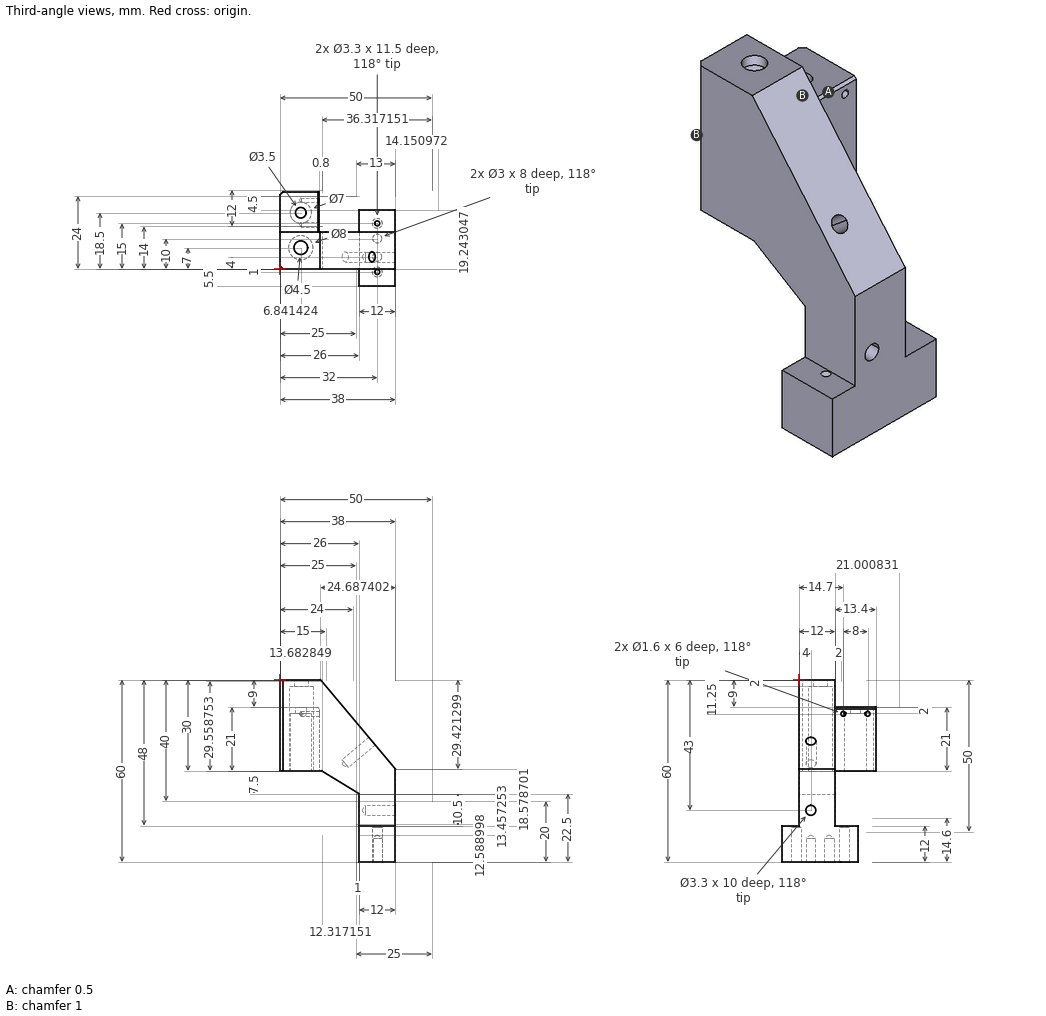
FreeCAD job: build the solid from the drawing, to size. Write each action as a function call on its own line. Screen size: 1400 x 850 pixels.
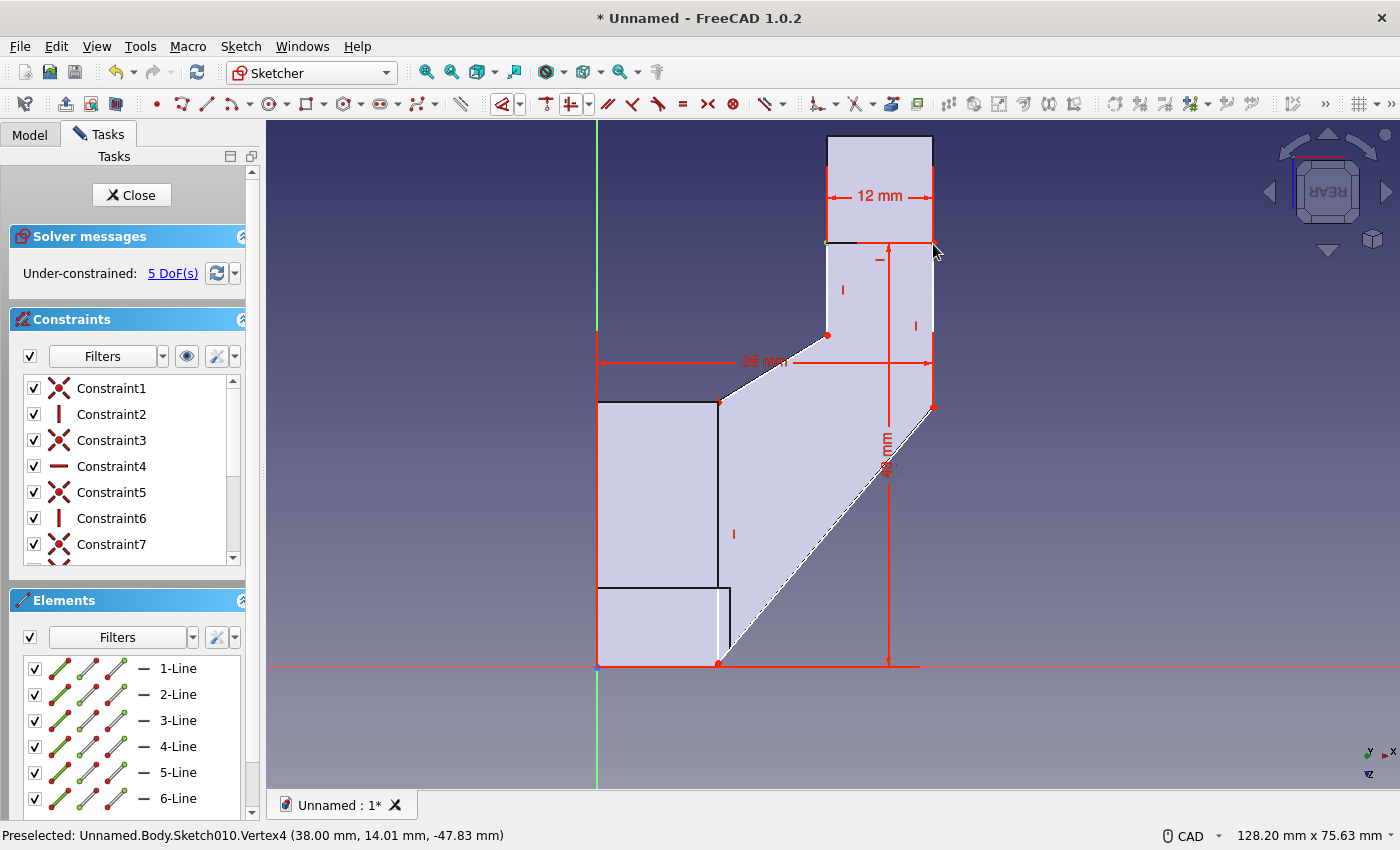
click(718, 403)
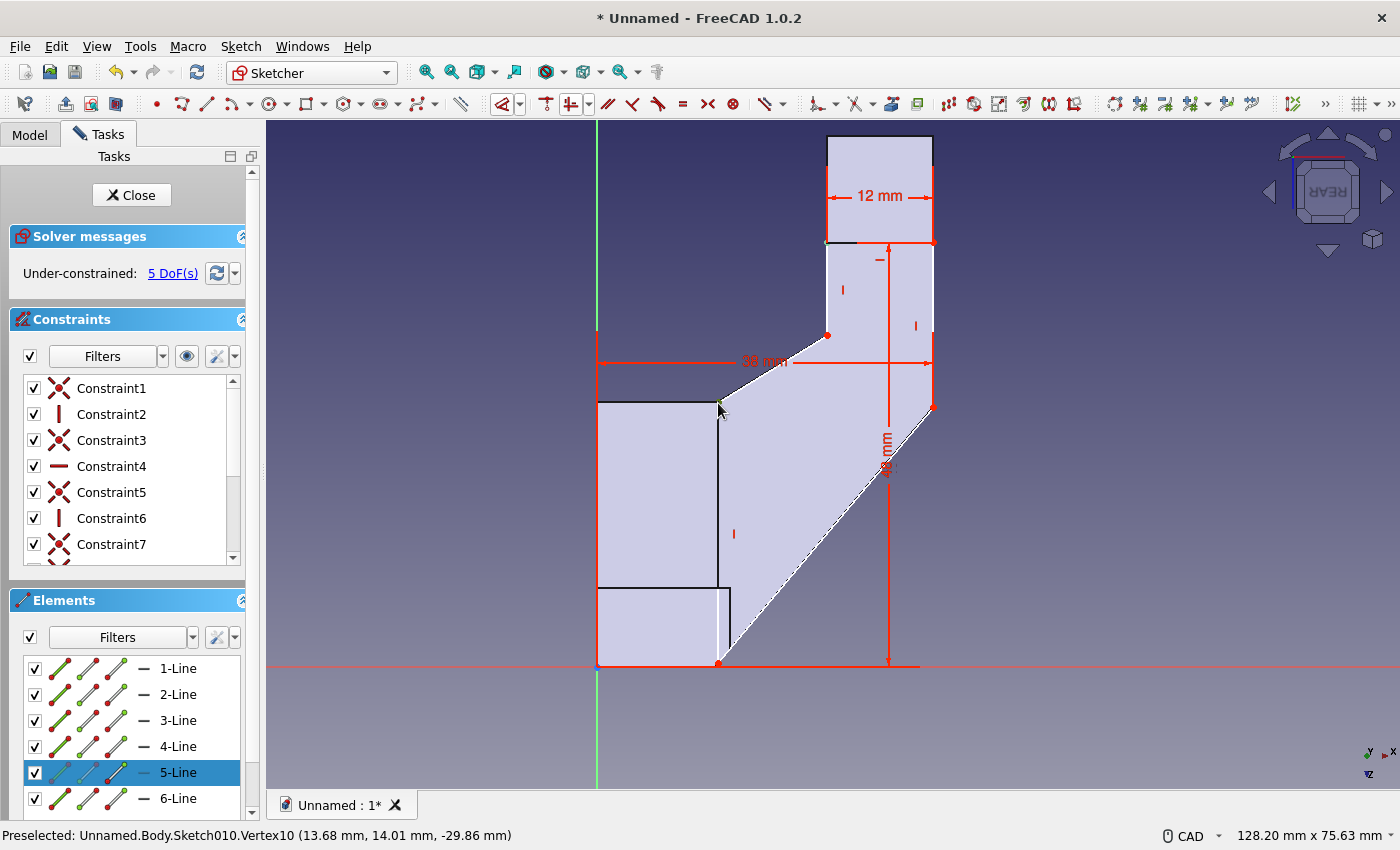
click(520, 104)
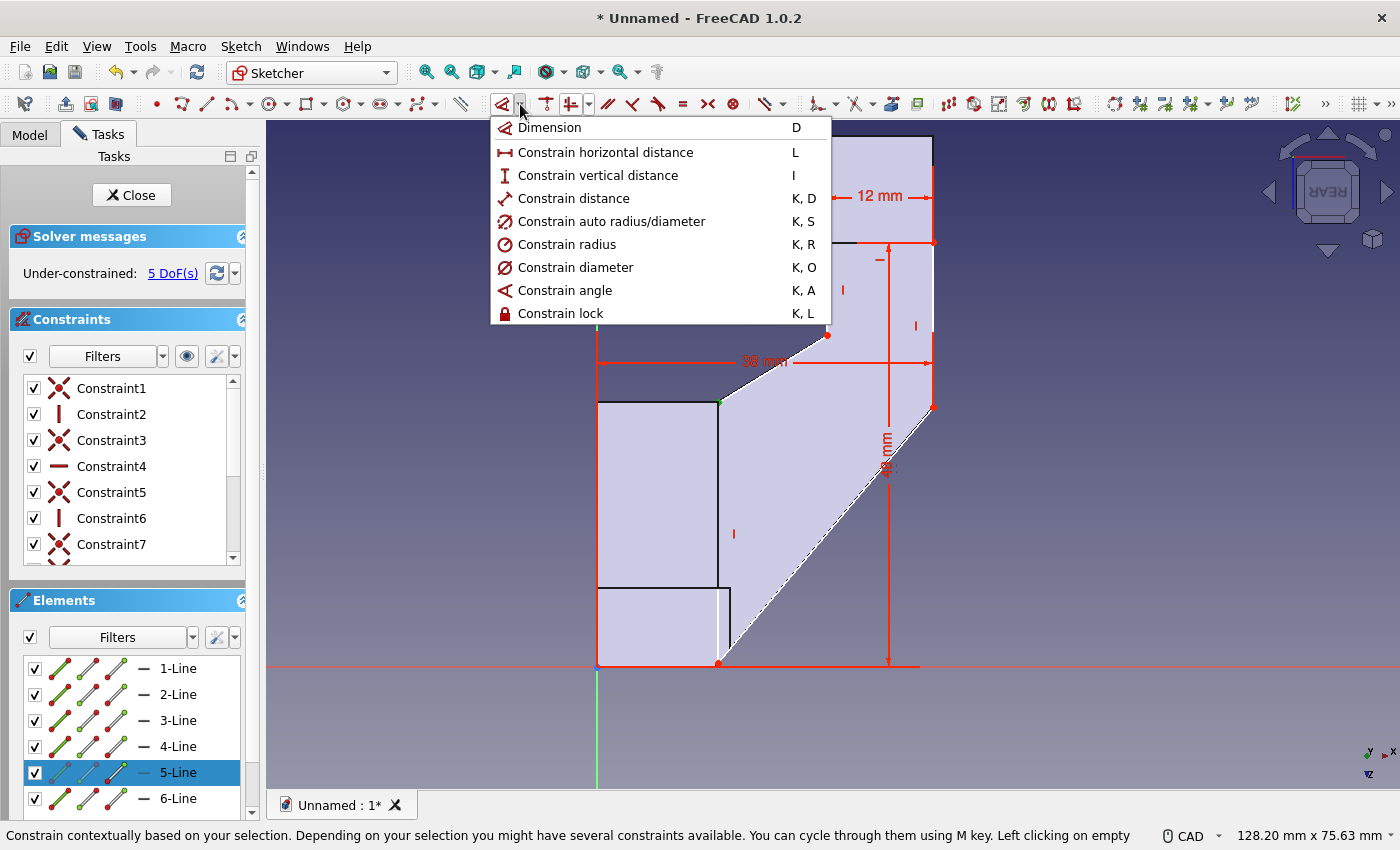
click(661, 176)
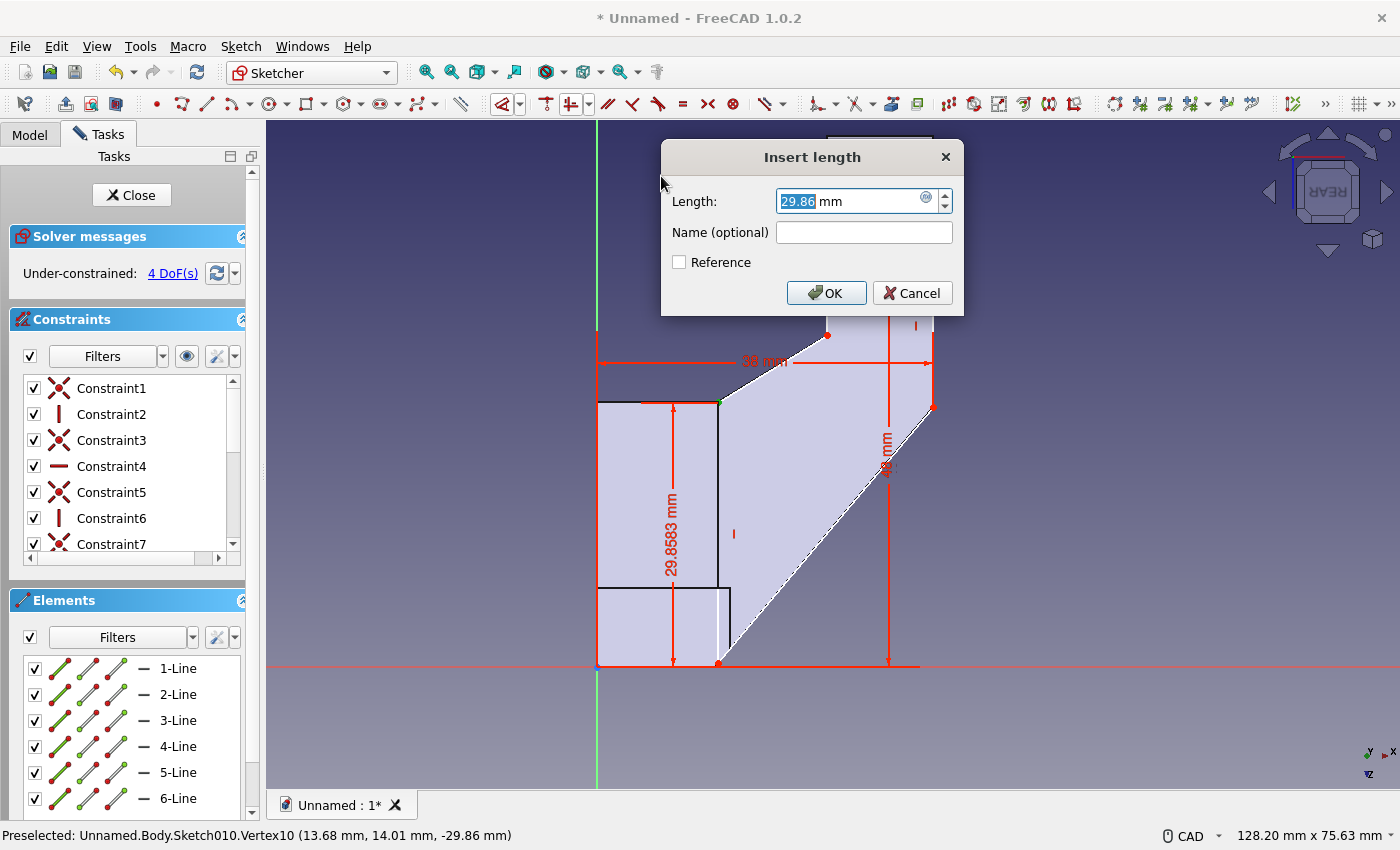
text(30)
key(Return)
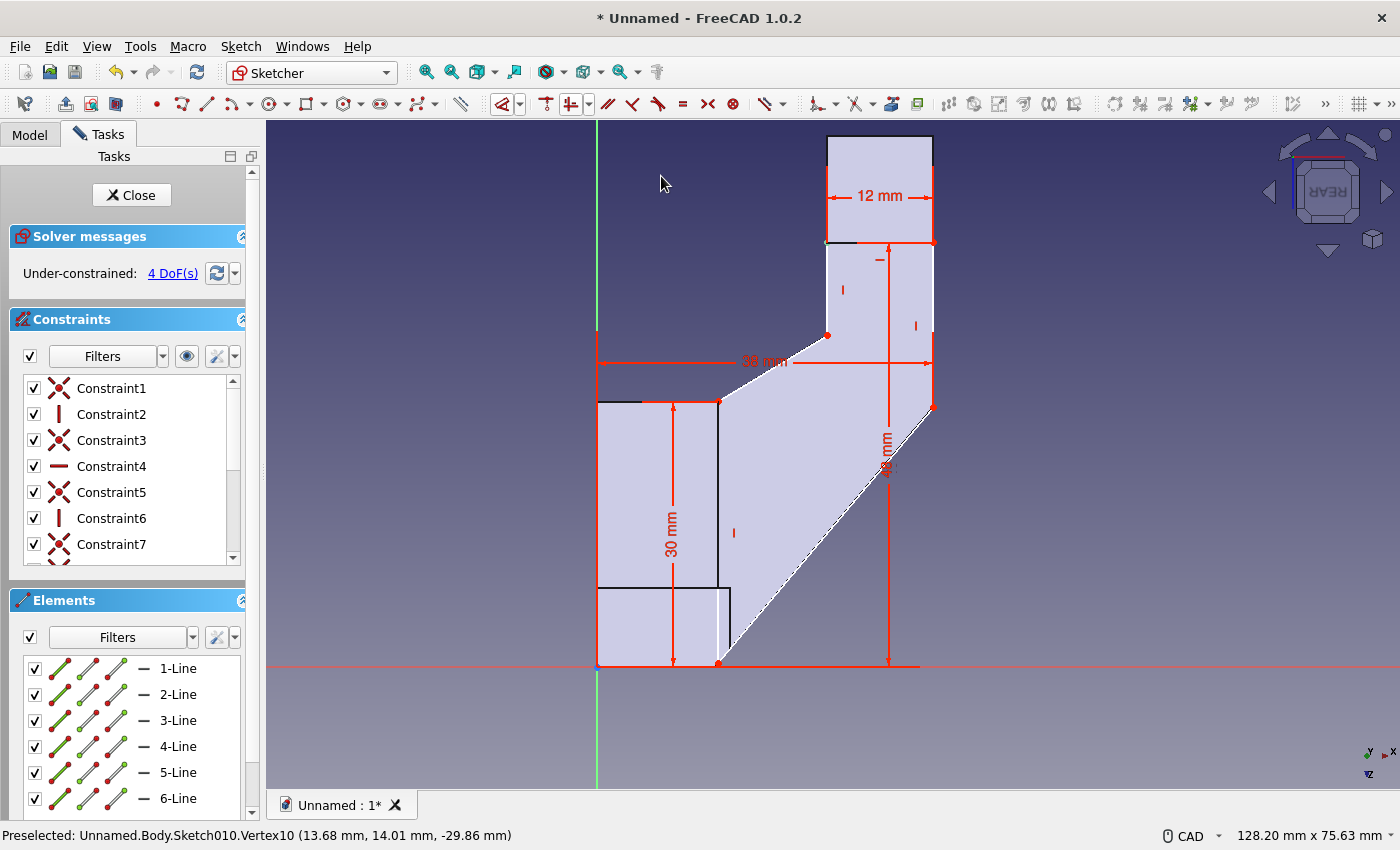
click(827, 271)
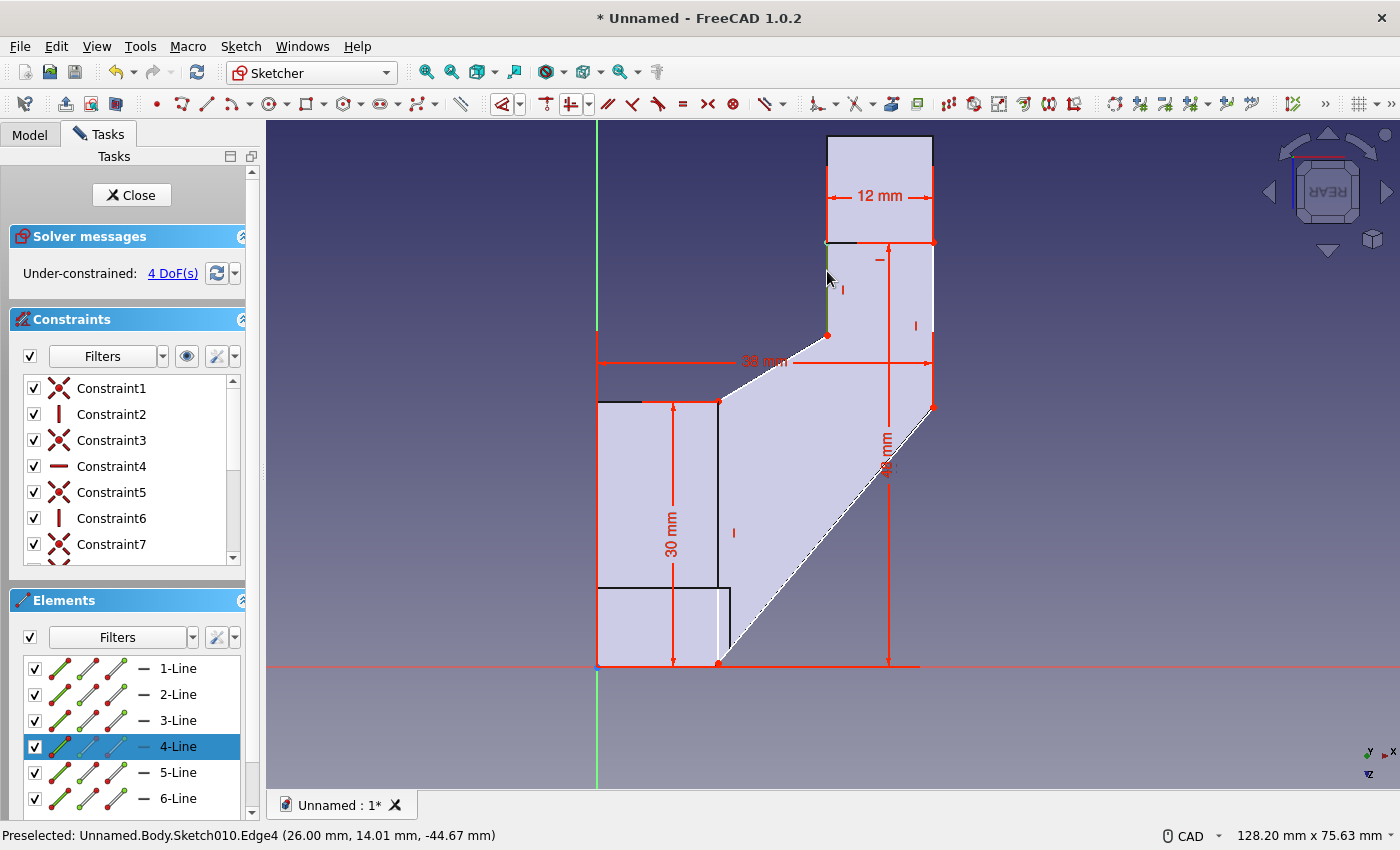
key(i)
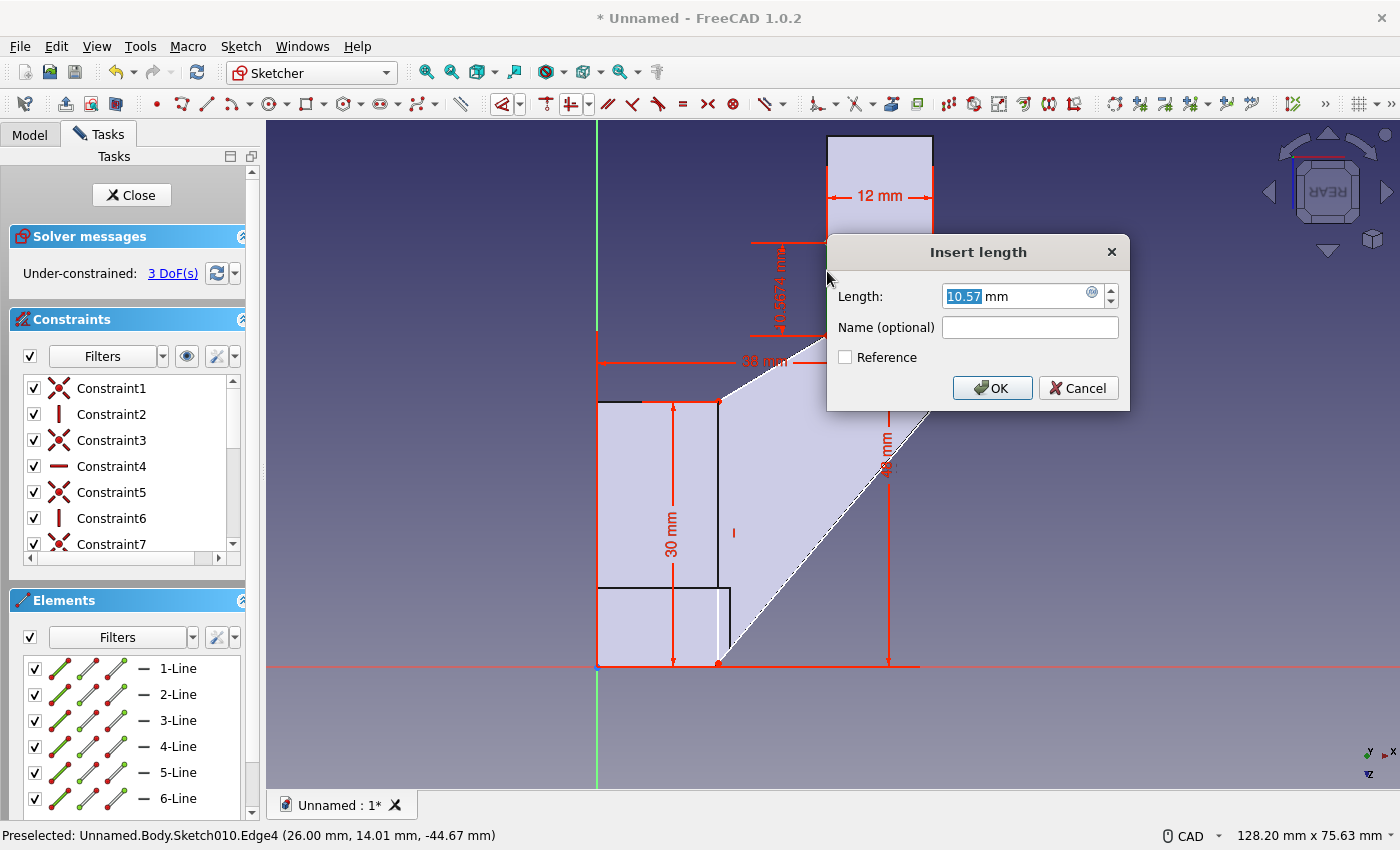
text(10.5)
key(Return)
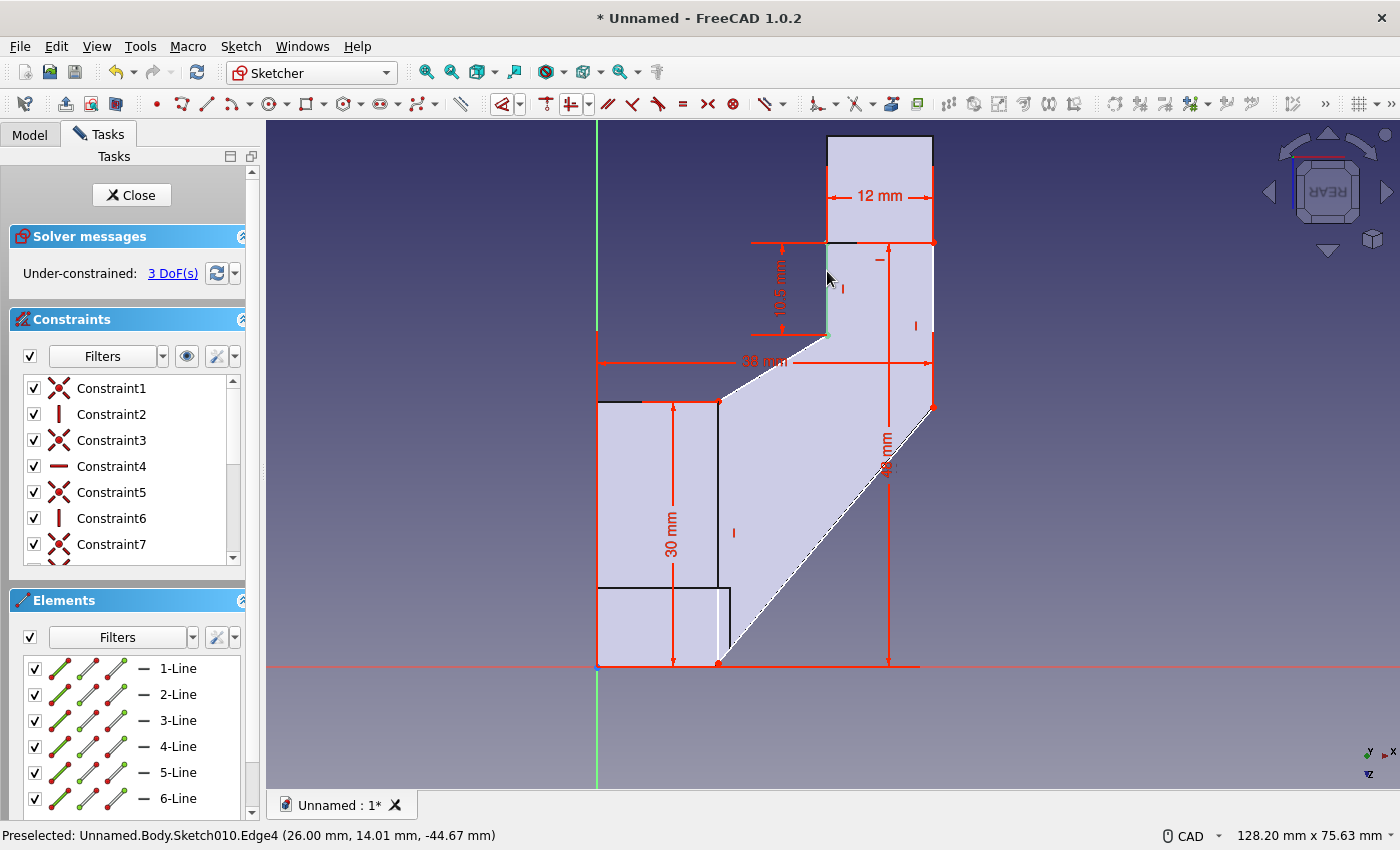
click(933, 358)